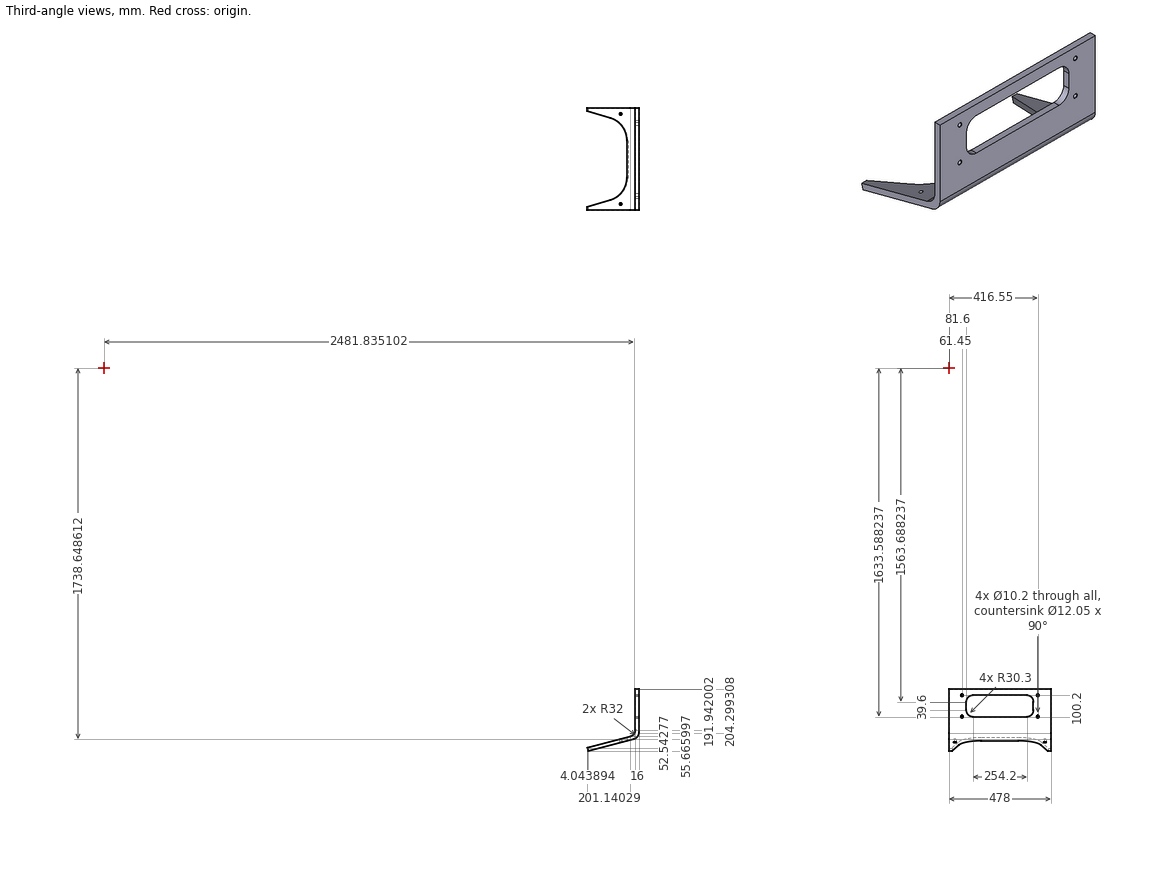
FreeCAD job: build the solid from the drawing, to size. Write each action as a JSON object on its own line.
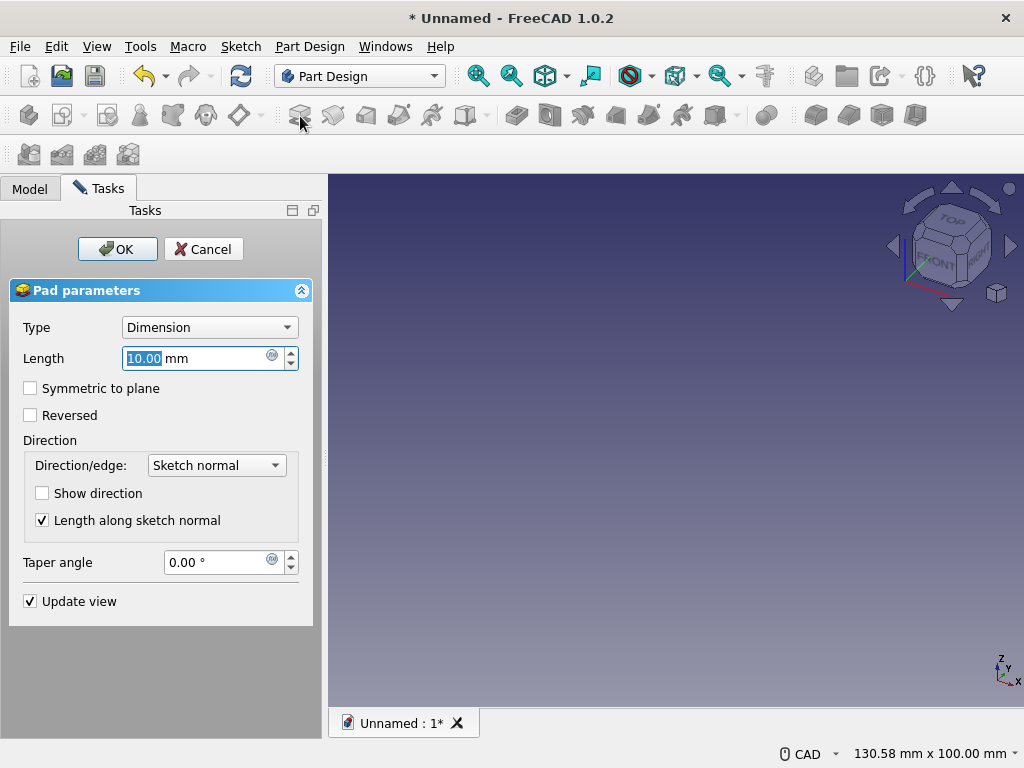
{"action": "type", "text": "478"}
{"action": "key", "text": "Tab"}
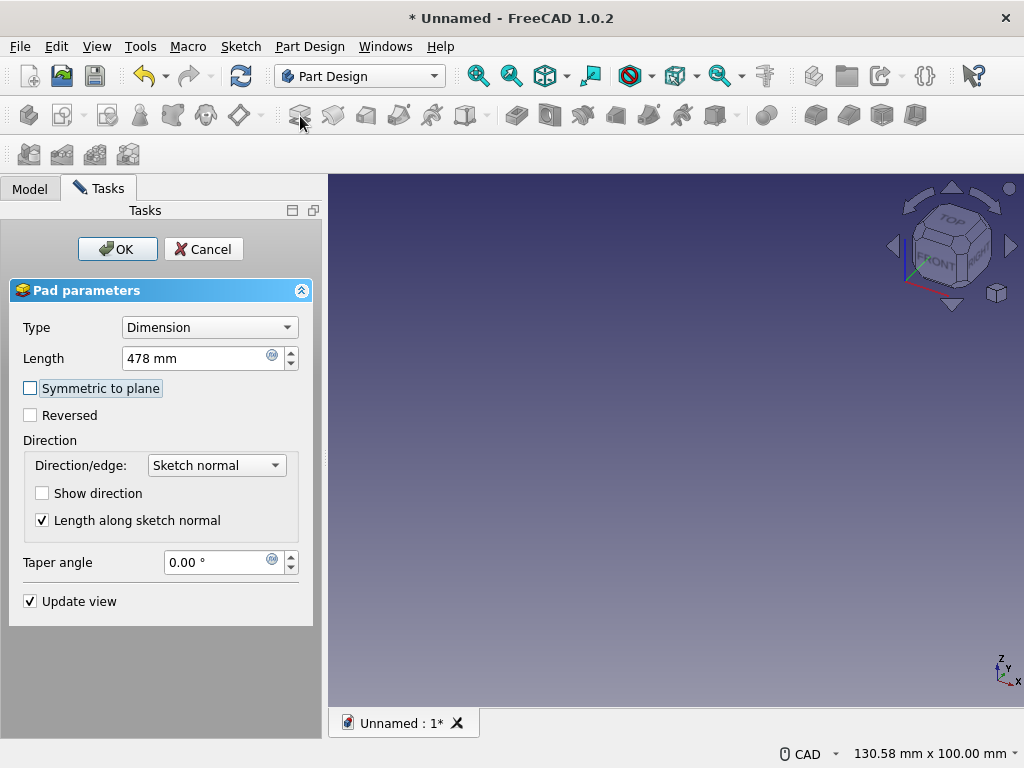
{"action": "left_click", "coordinate": [31, 415]}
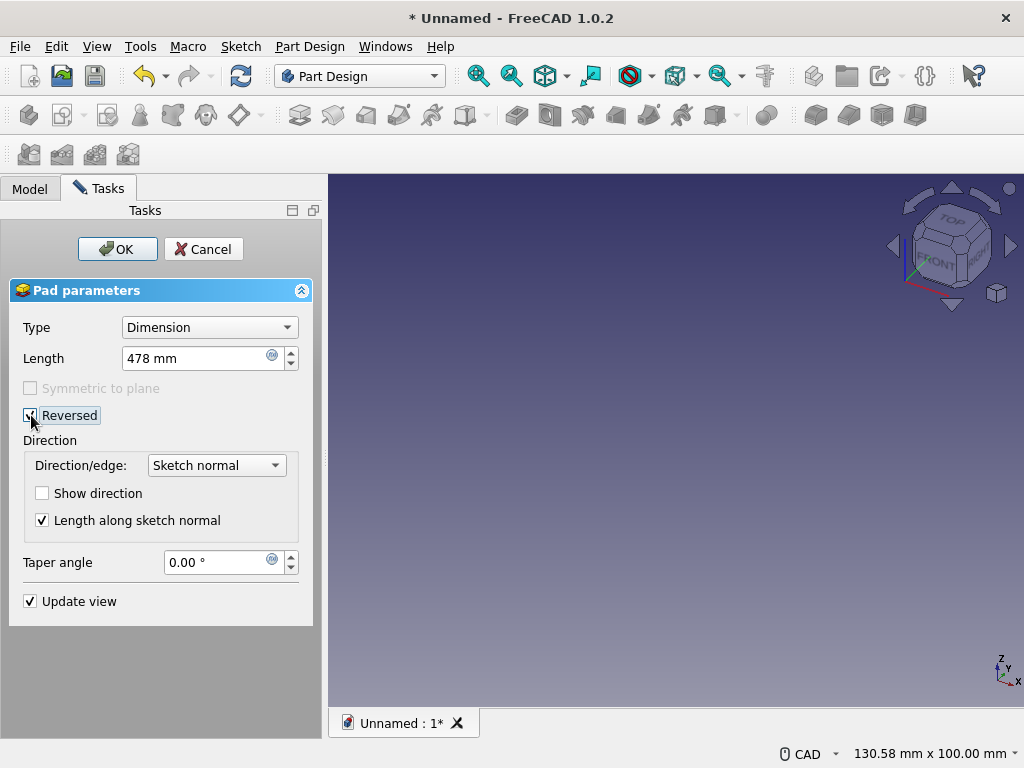
{"action": "left_click", "coordinate": [118, 249]}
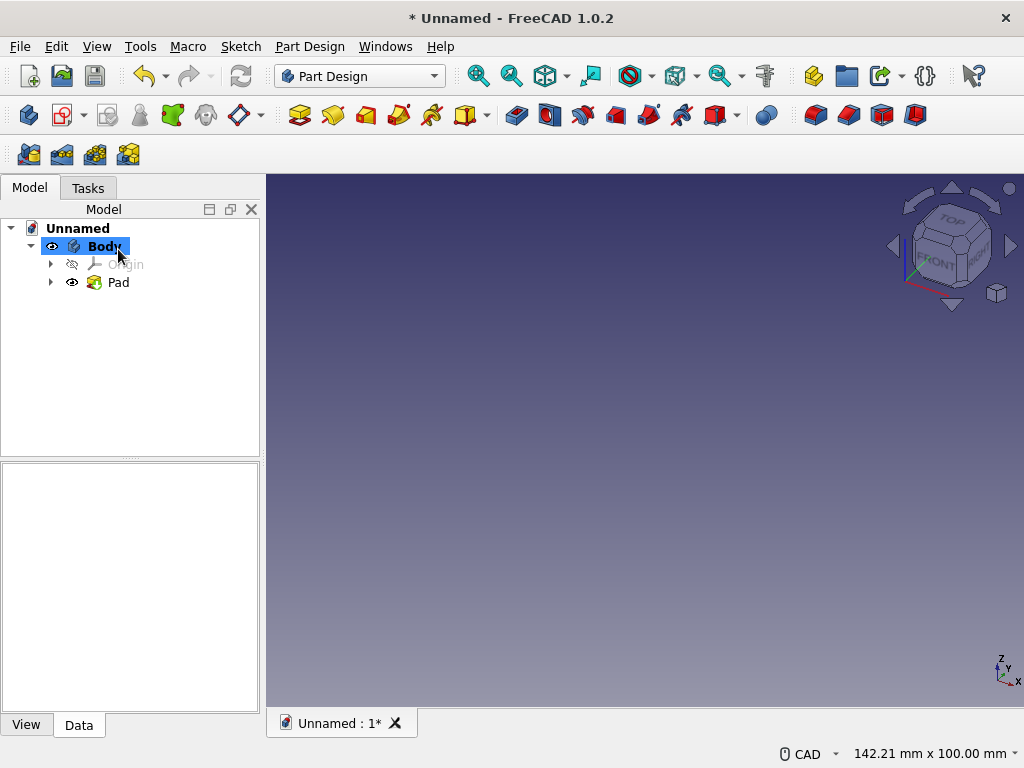
{"action": "left_click", "coordinate": [479, 76]}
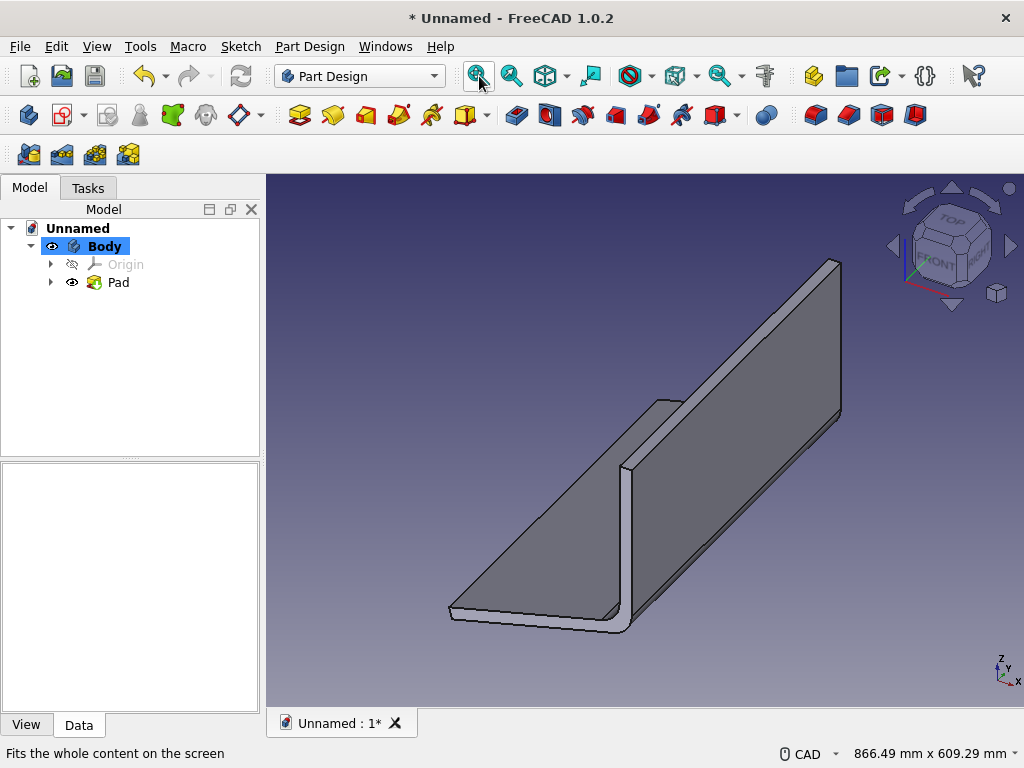
{"action": "left_click", "coordinate": [736, 439]}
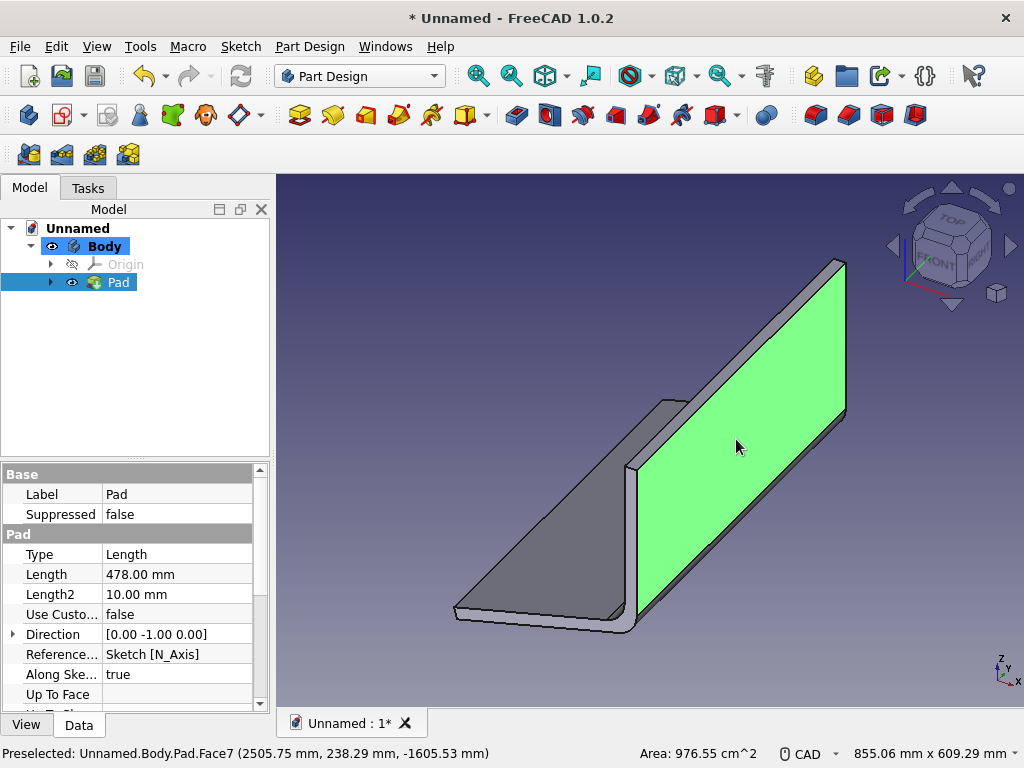
{"action": "left_click", "coordinate": [62, 116]}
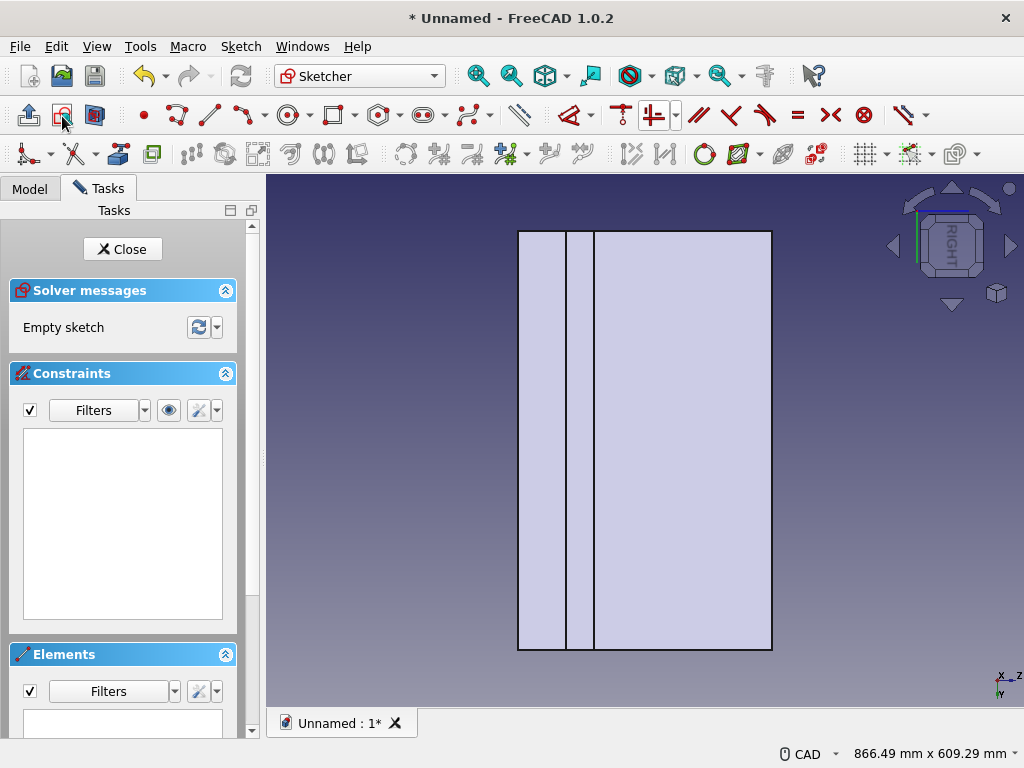
{"action": "left_click", "coordinate": [210, 116]}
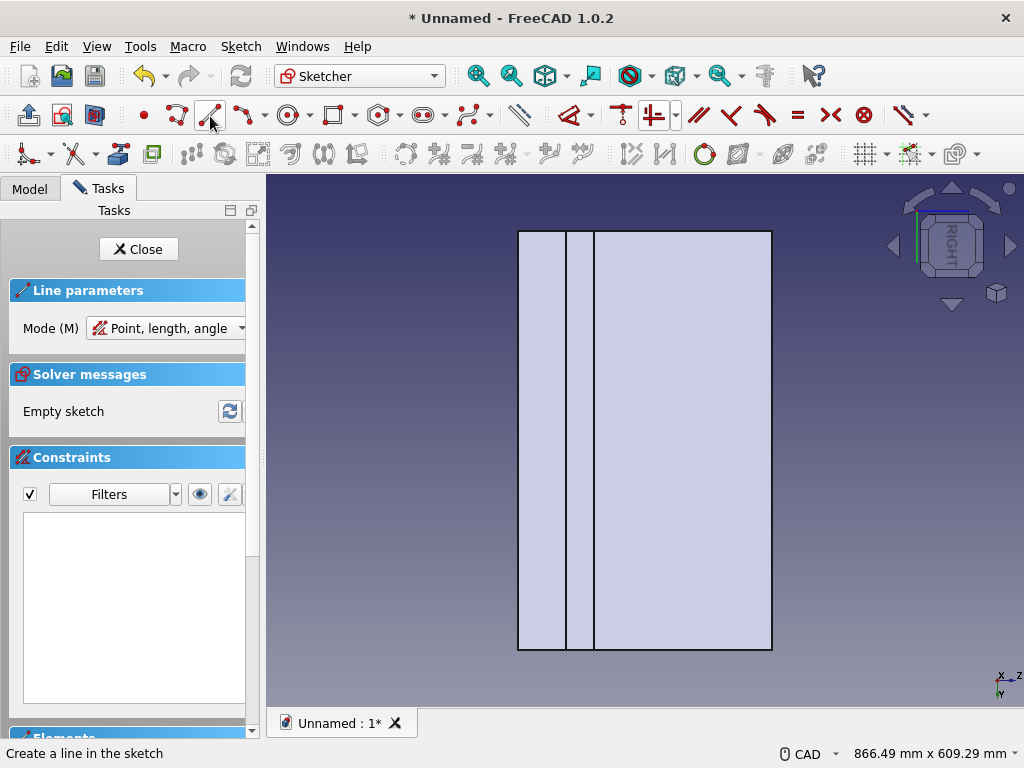
{"action": "left_click", "coordinate": [720, 303]}
{"action": "left_click", "coordinate": [685, 303]}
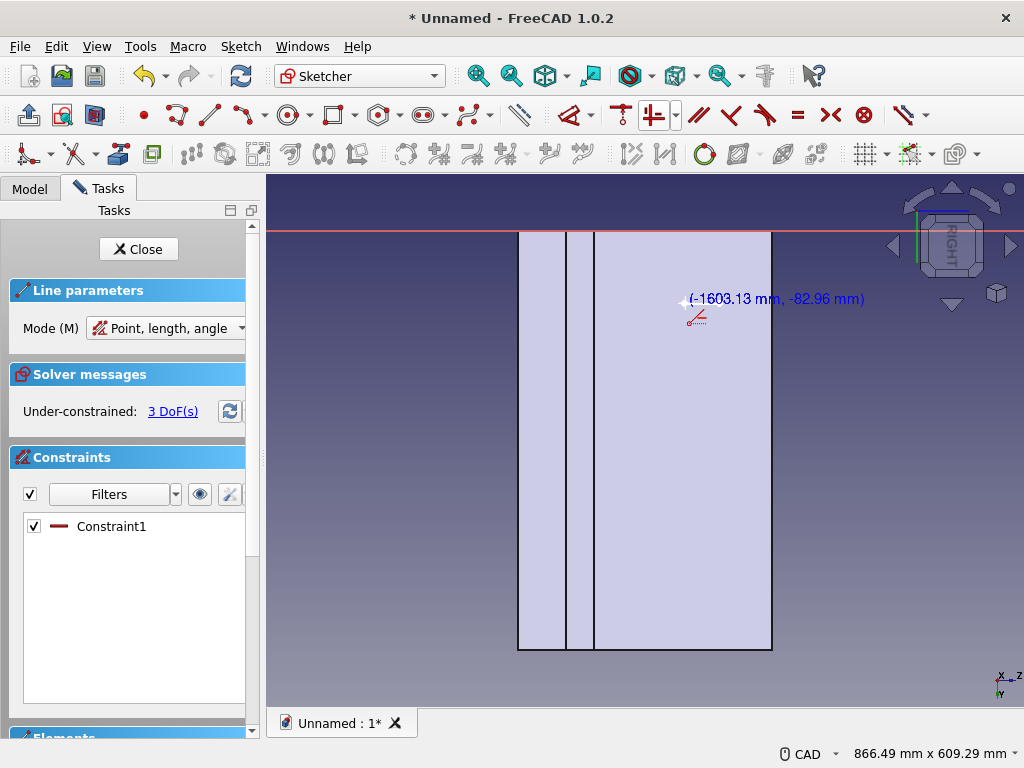
{"action": "left_click", "coordinate": [658, 329]}
{"action": "left_click", "coordinate": [658, 552]}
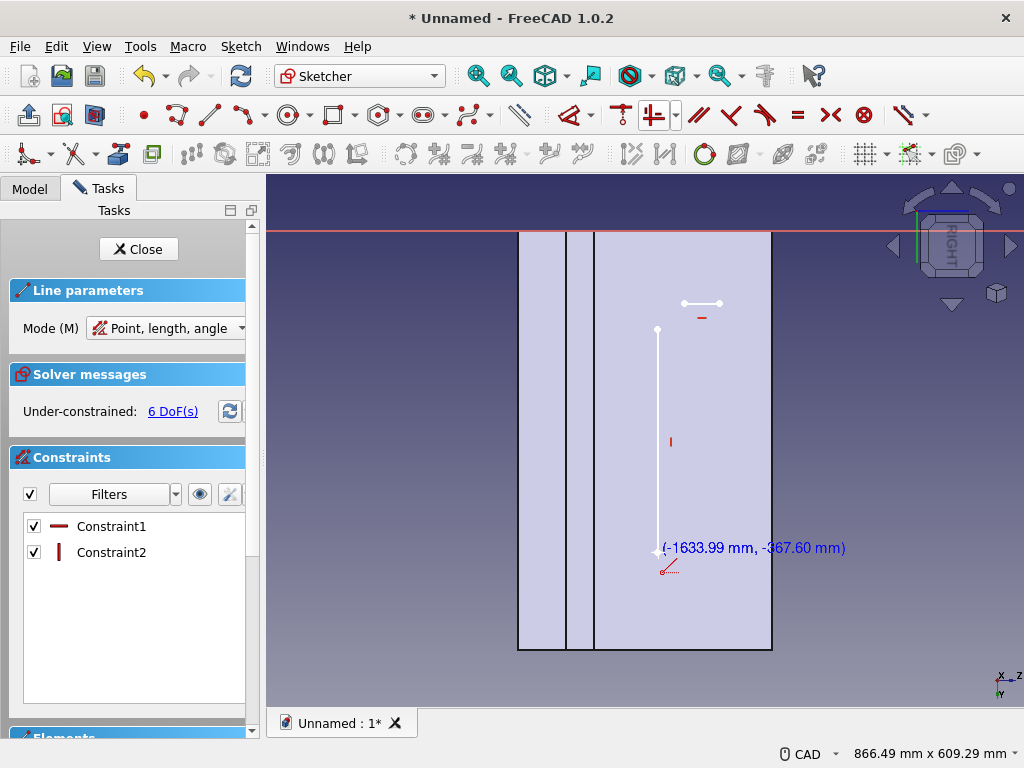
{"action": "left_click", "coordinate": [685, 578]}
{"action": "left_click", "coordinate": [720, 578]}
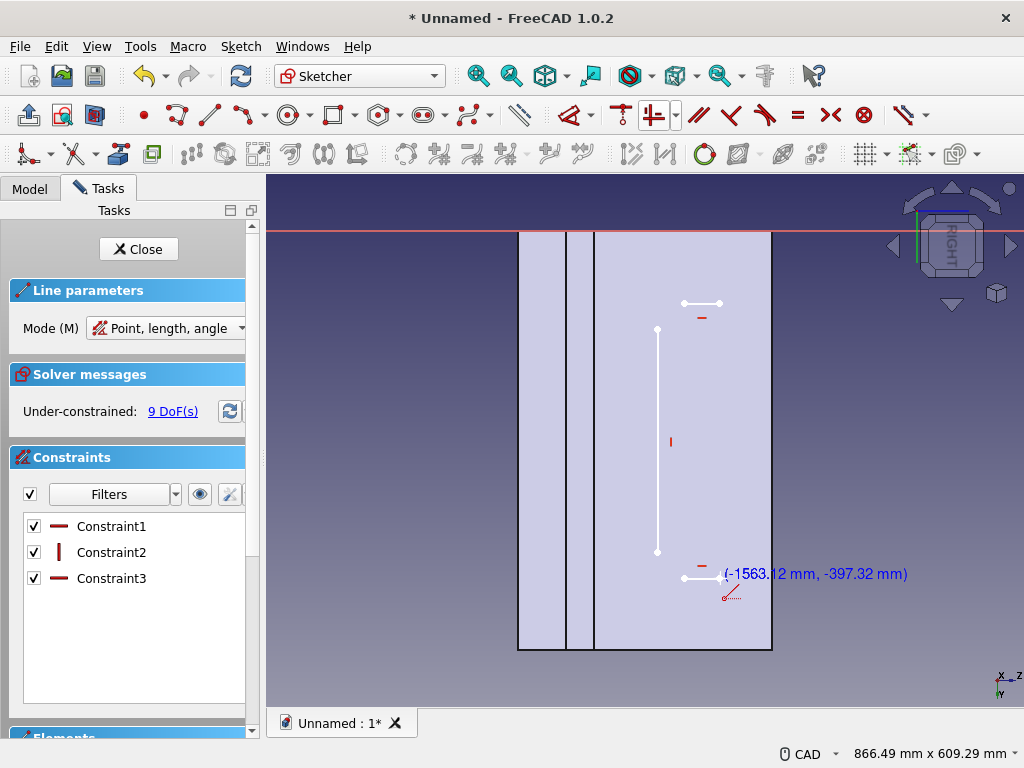
{"action": "left_click", "coordinate": [746, 552]}
{"action": "left_click", "coordinate": [746, 329]}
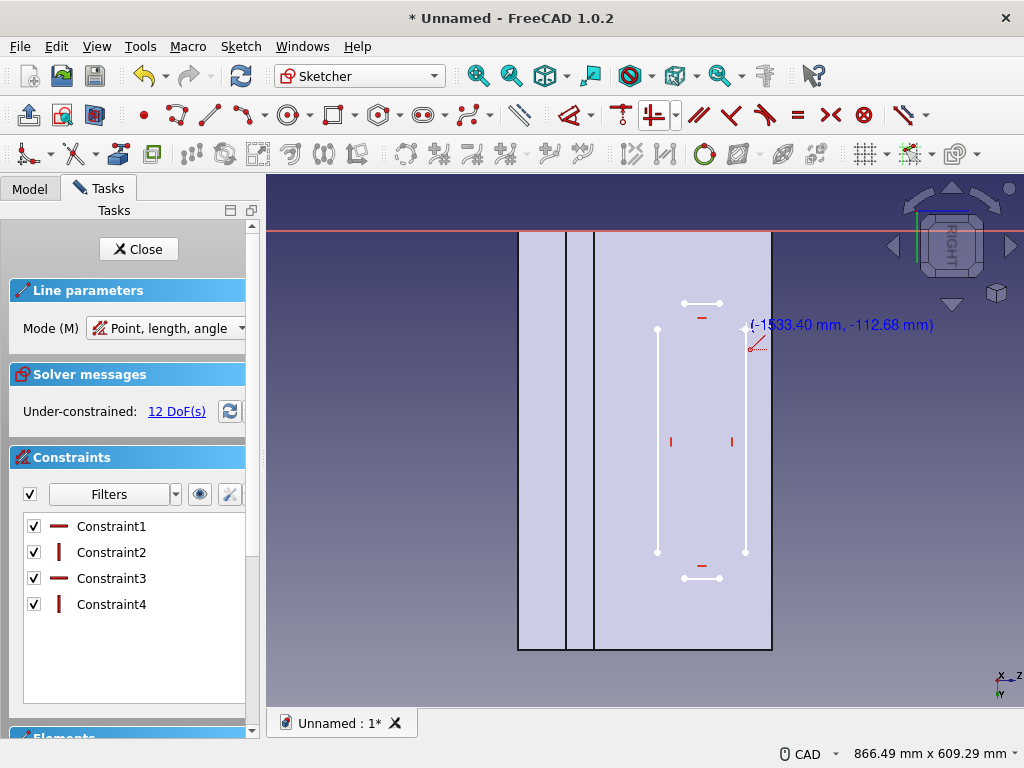
{"action": "left_click", "coordinate": [242, 116]}